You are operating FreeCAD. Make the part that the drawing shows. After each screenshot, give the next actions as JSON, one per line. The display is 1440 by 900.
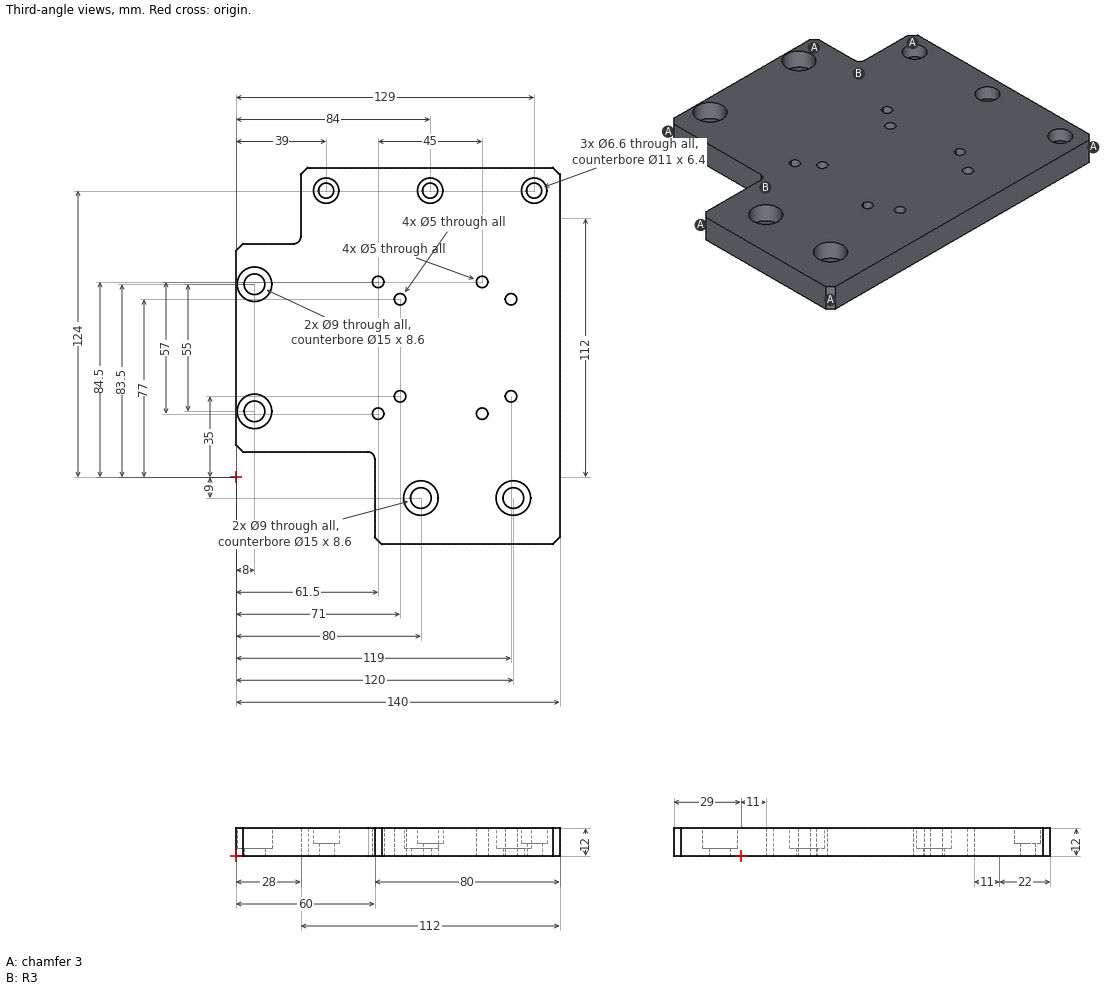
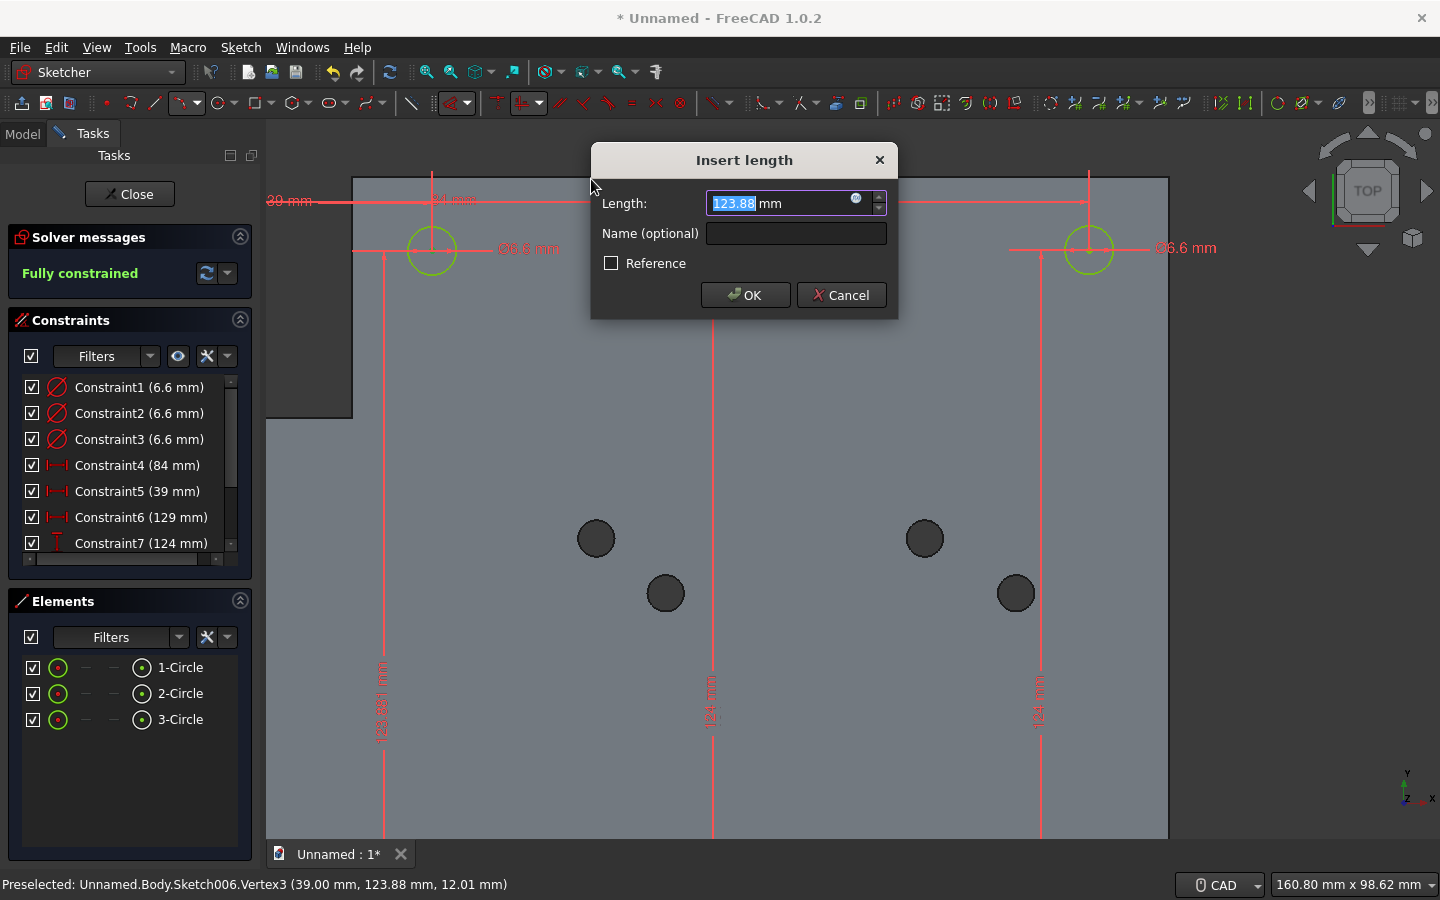
{"action": "type", "text": "124"}
{"action": "key", "text": "Return"}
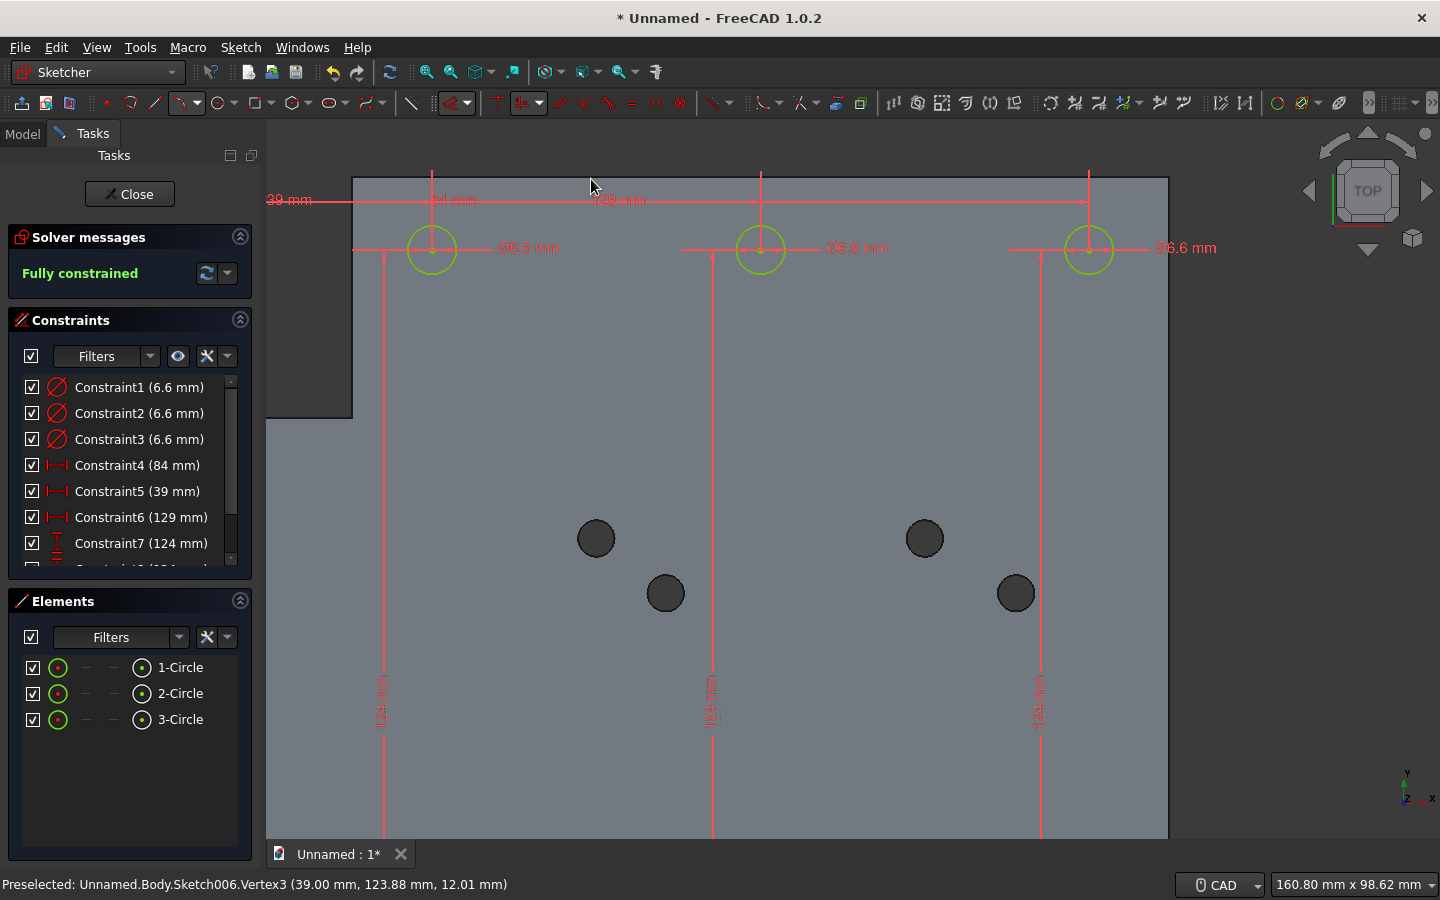
{"action": "left_click", "coordinate": [130, 194]}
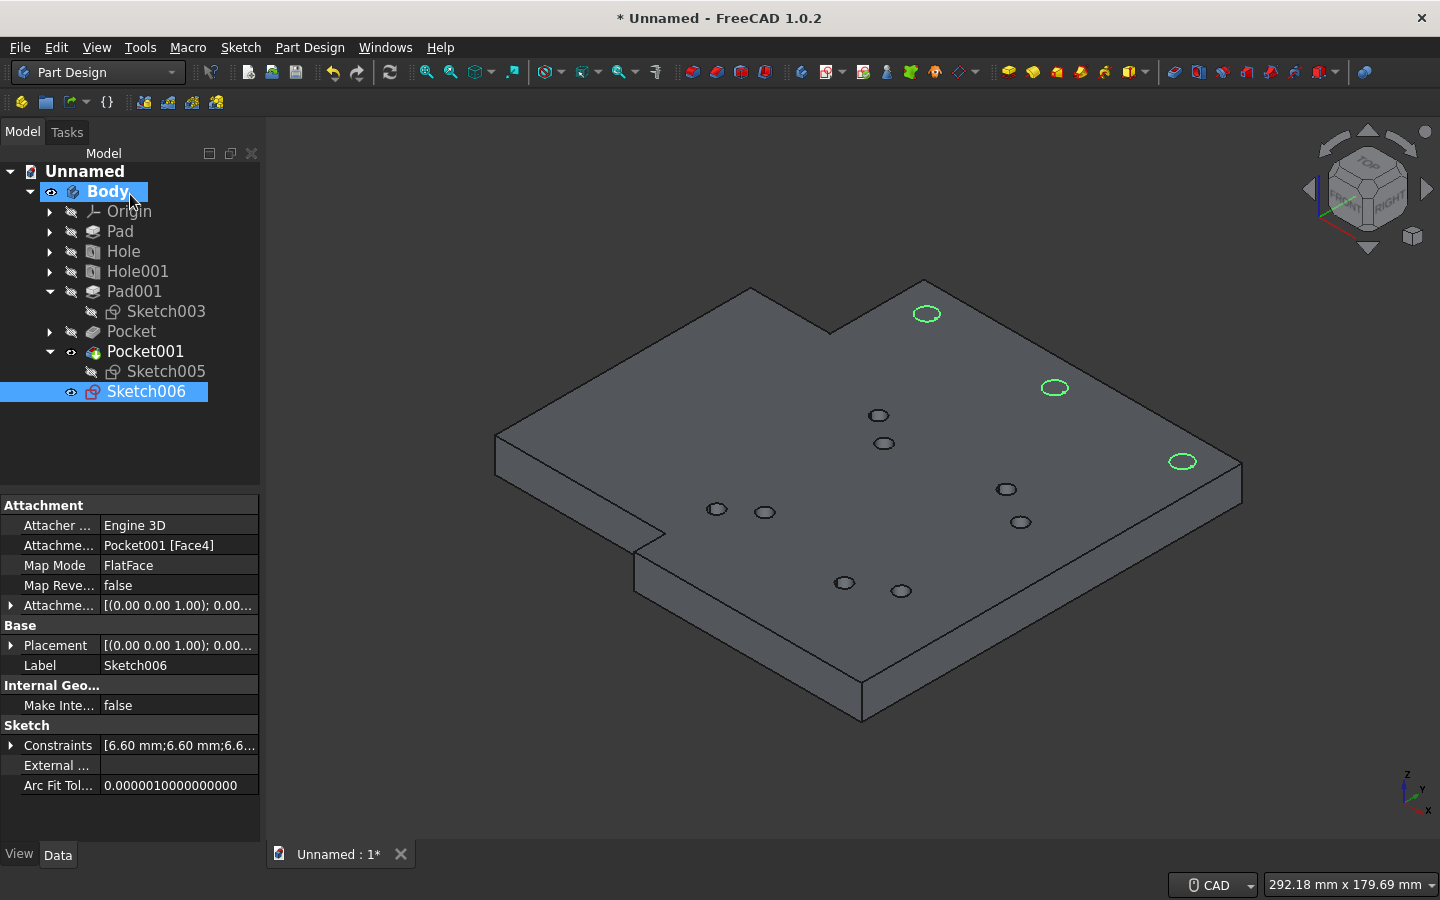
{"action": "left_click", "coordinate": [1200, 72]}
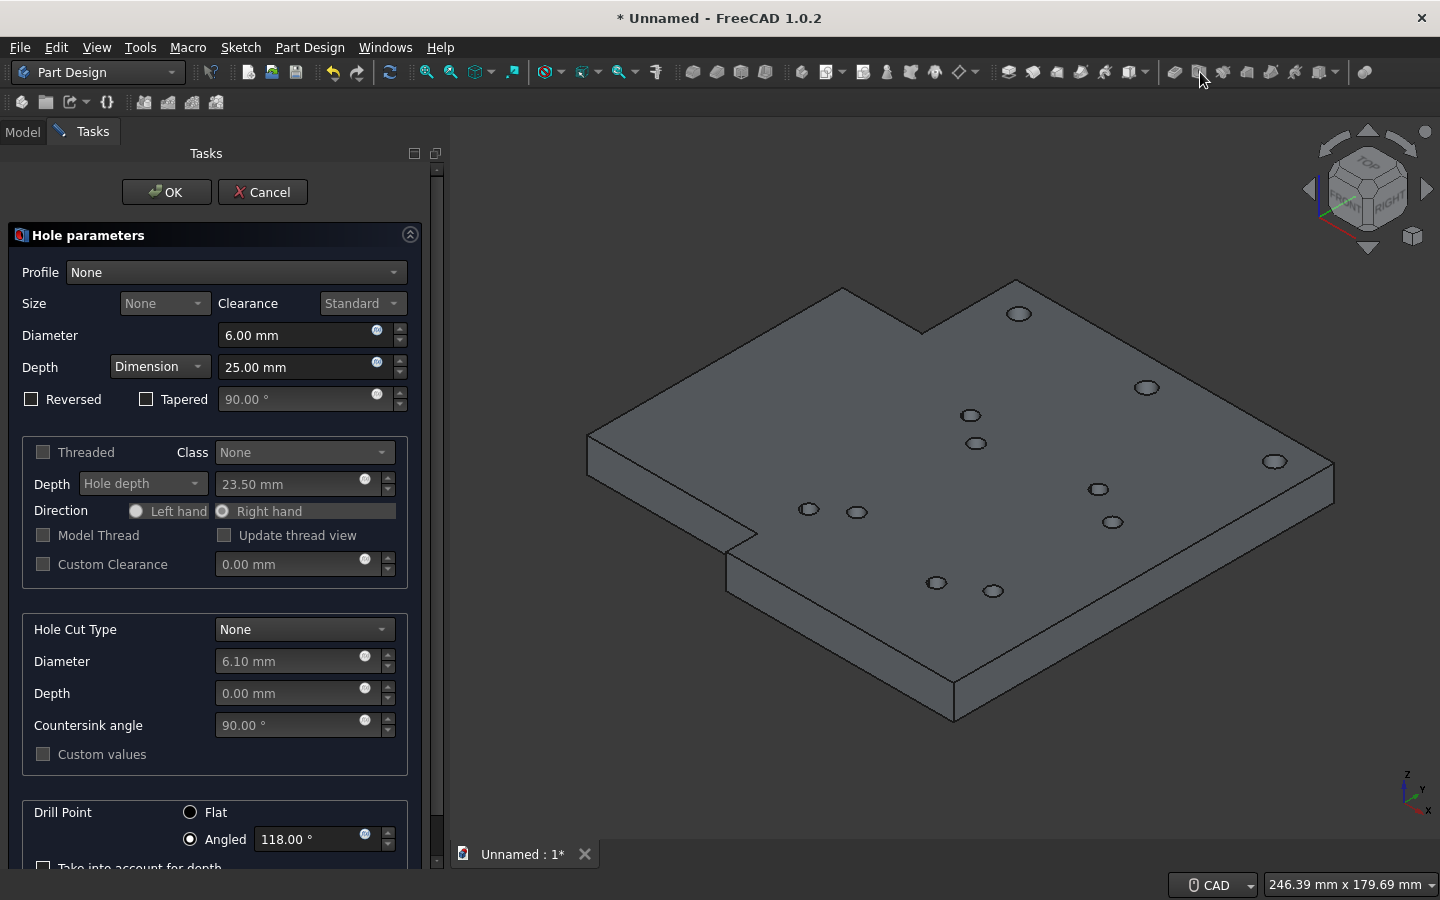
{"action": "triple_click", "coordinate": [305, 335]}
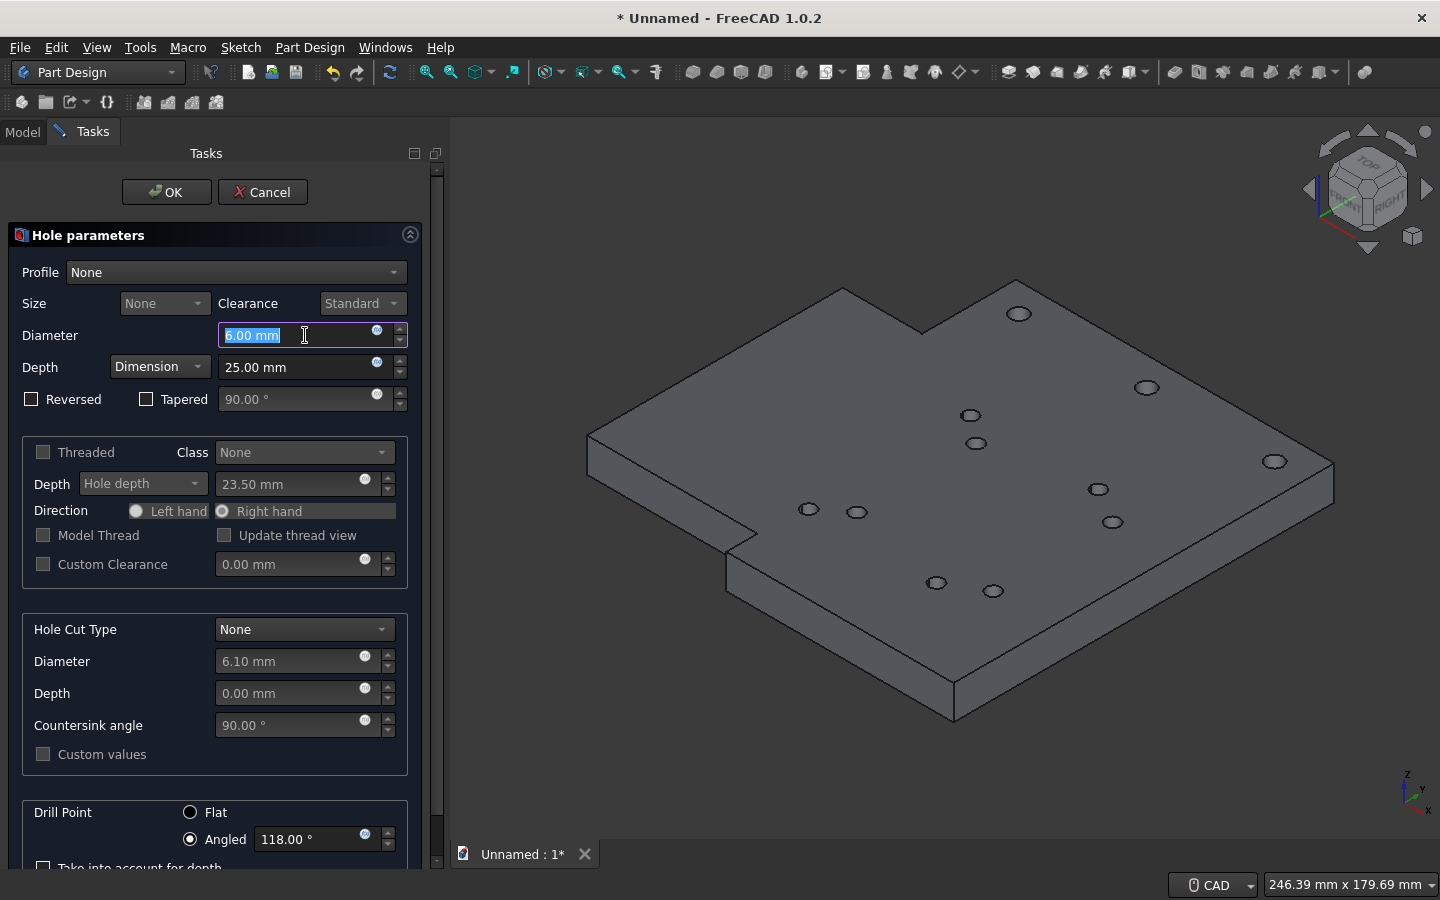
{"action": "type", "text": "6.6"}
{"action": "key", "text": "Tab"}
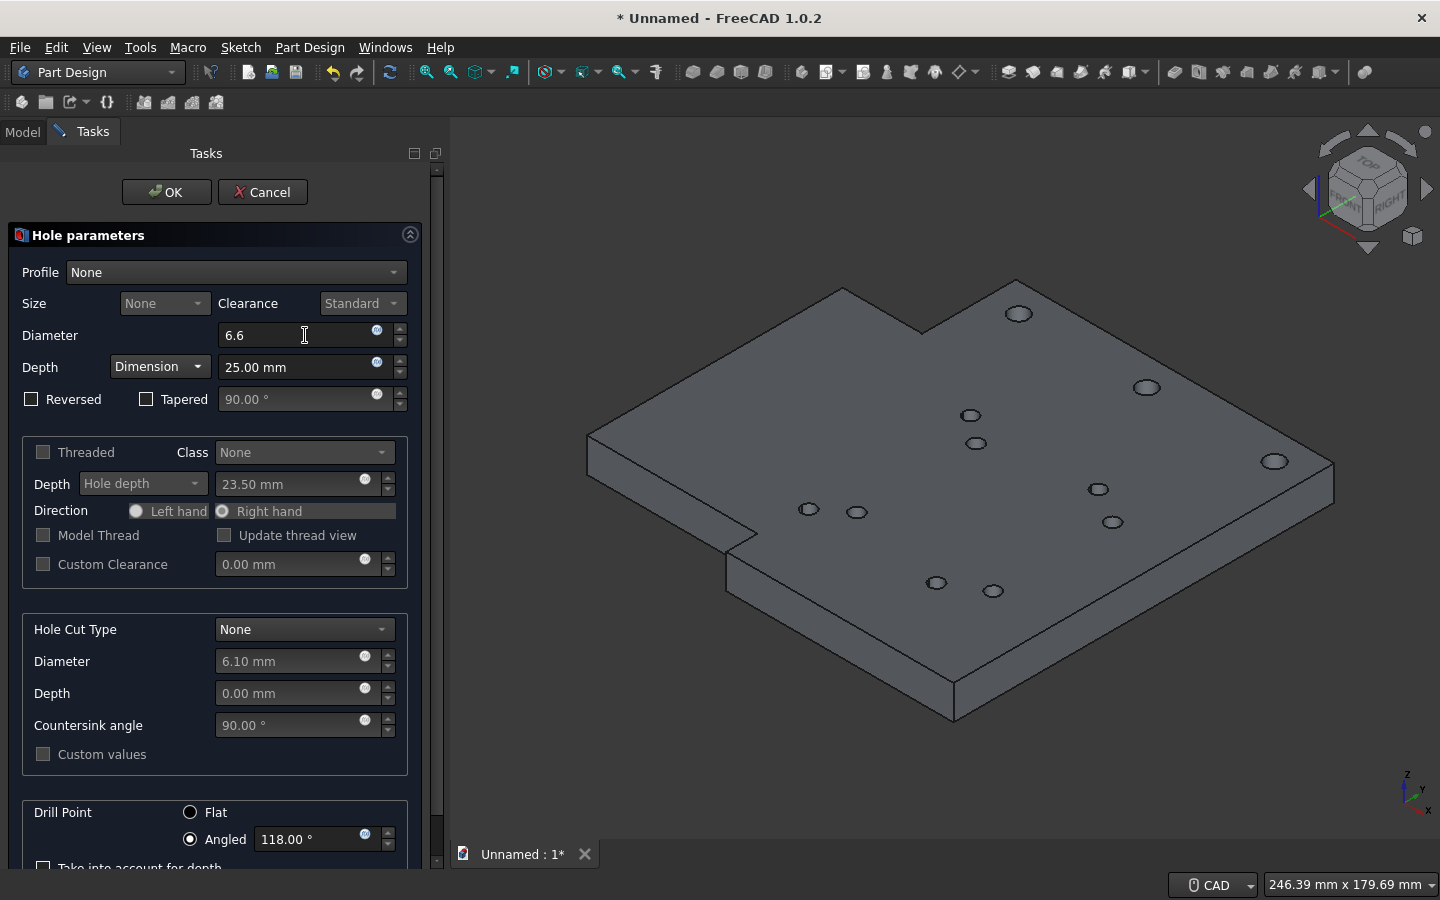
{"action": "left_click", "coordinate": [161, 366]}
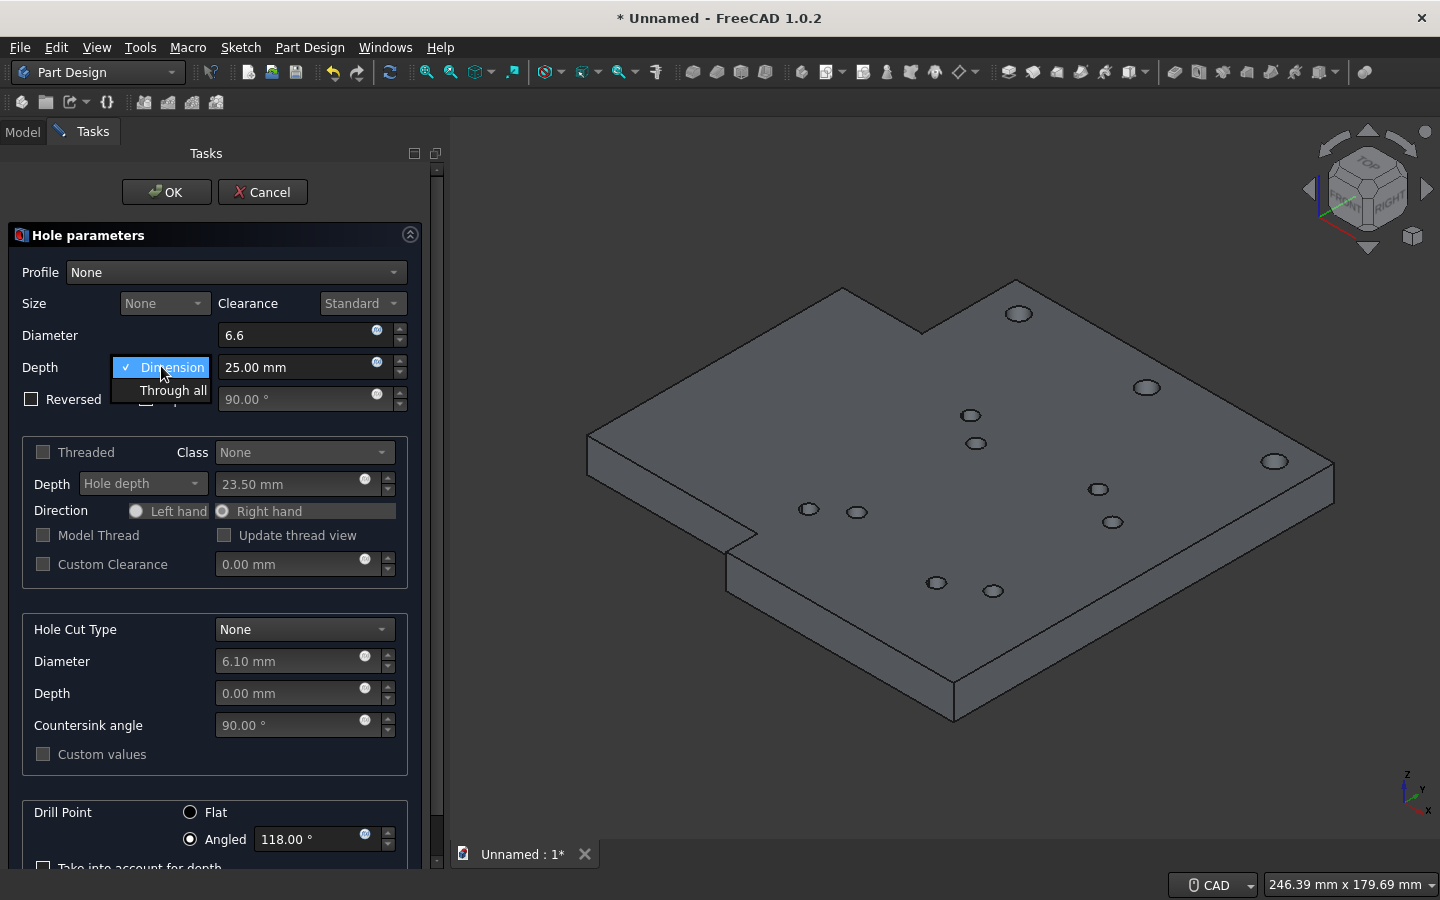
{"action": "left_click", "coordinate": [160, 390]}